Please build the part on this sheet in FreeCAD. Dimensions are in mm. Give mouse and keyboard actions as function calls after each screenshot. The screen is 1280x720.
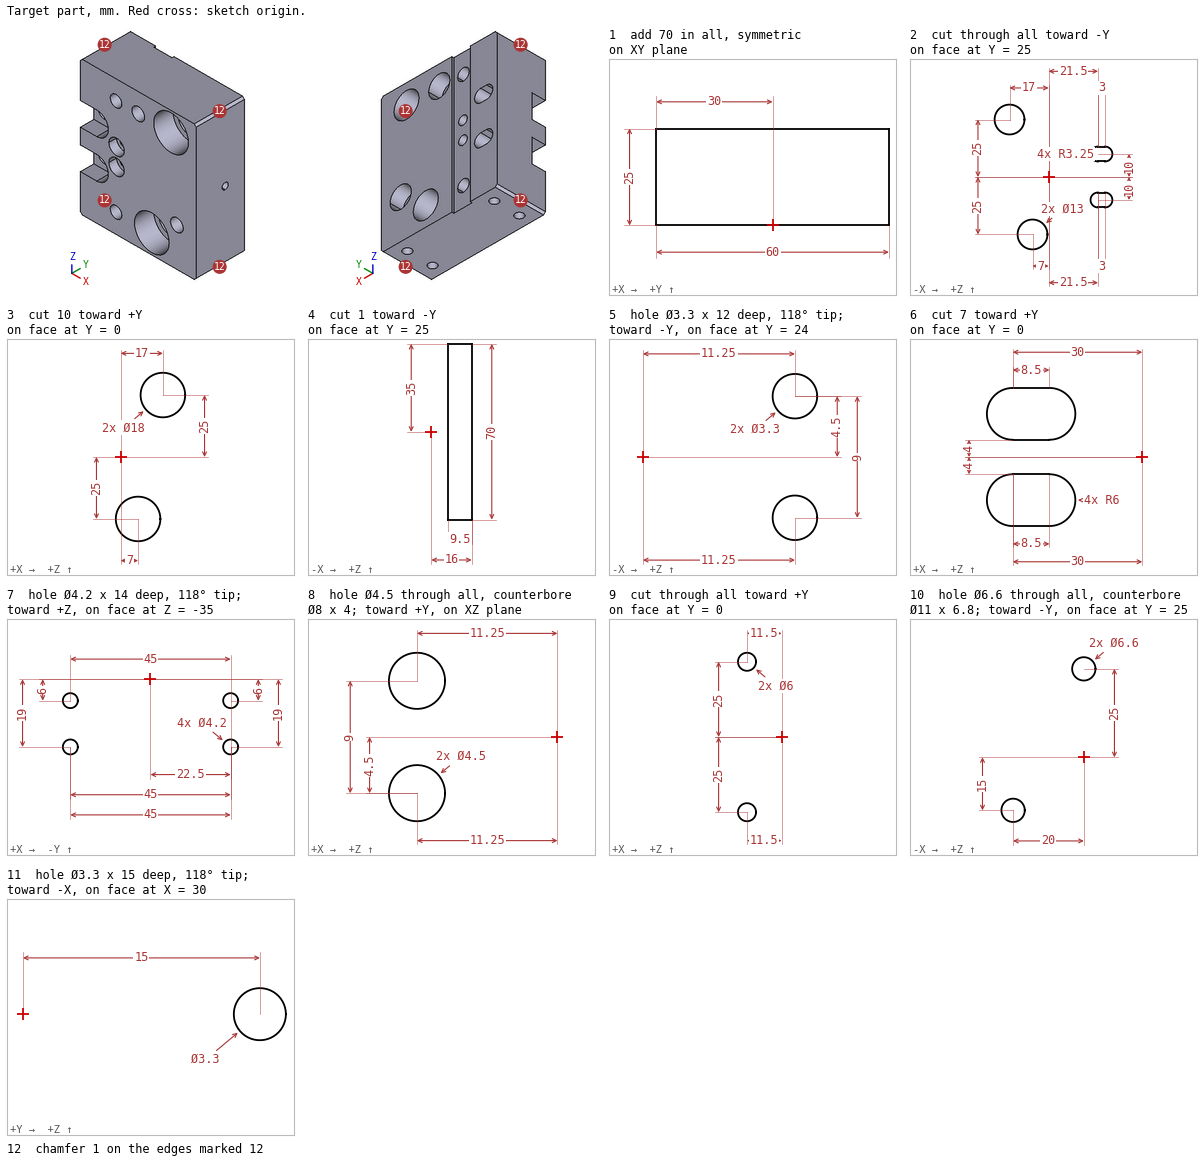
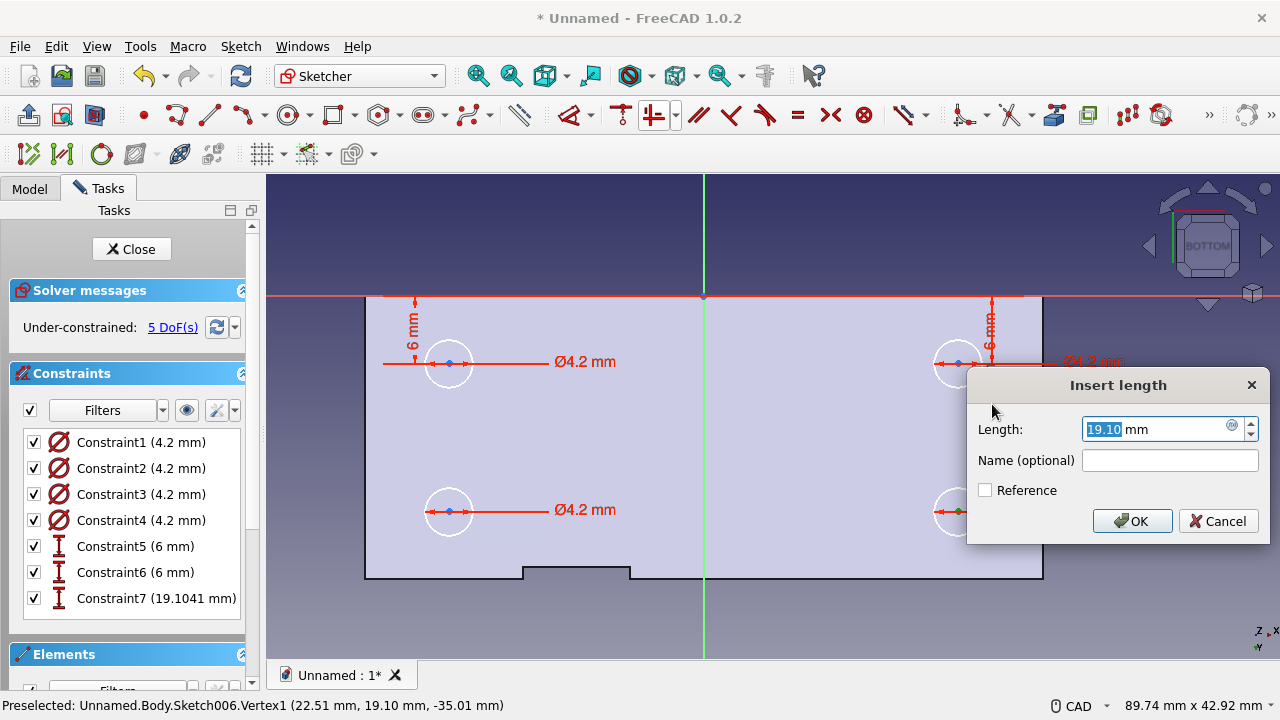
text(19)
key(Return)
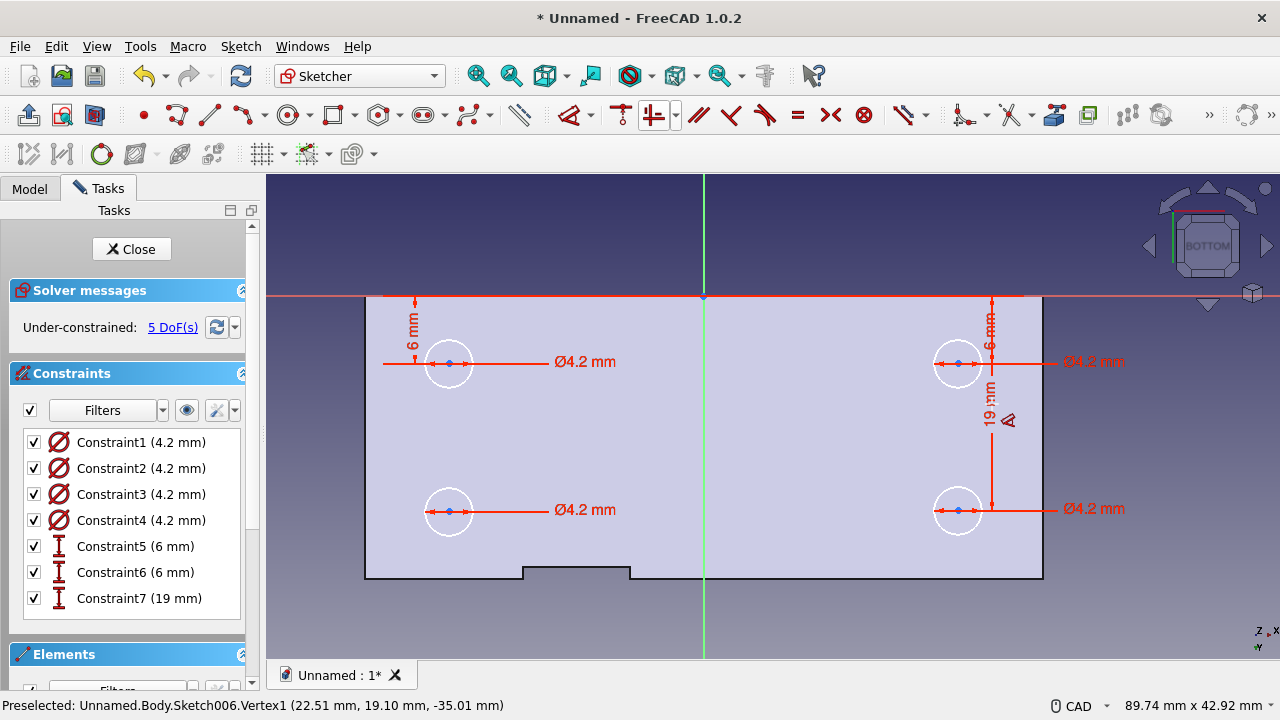
click(449, 512)
click(415, 404)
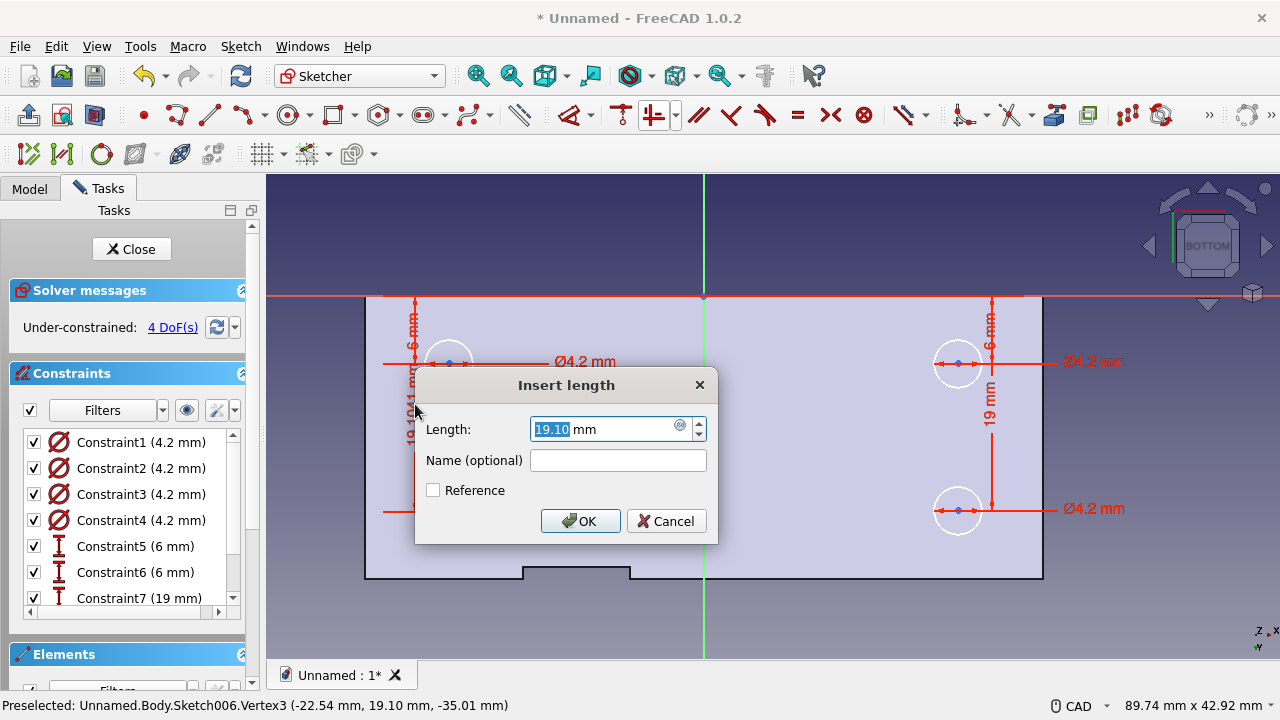
text(19)
key(Return)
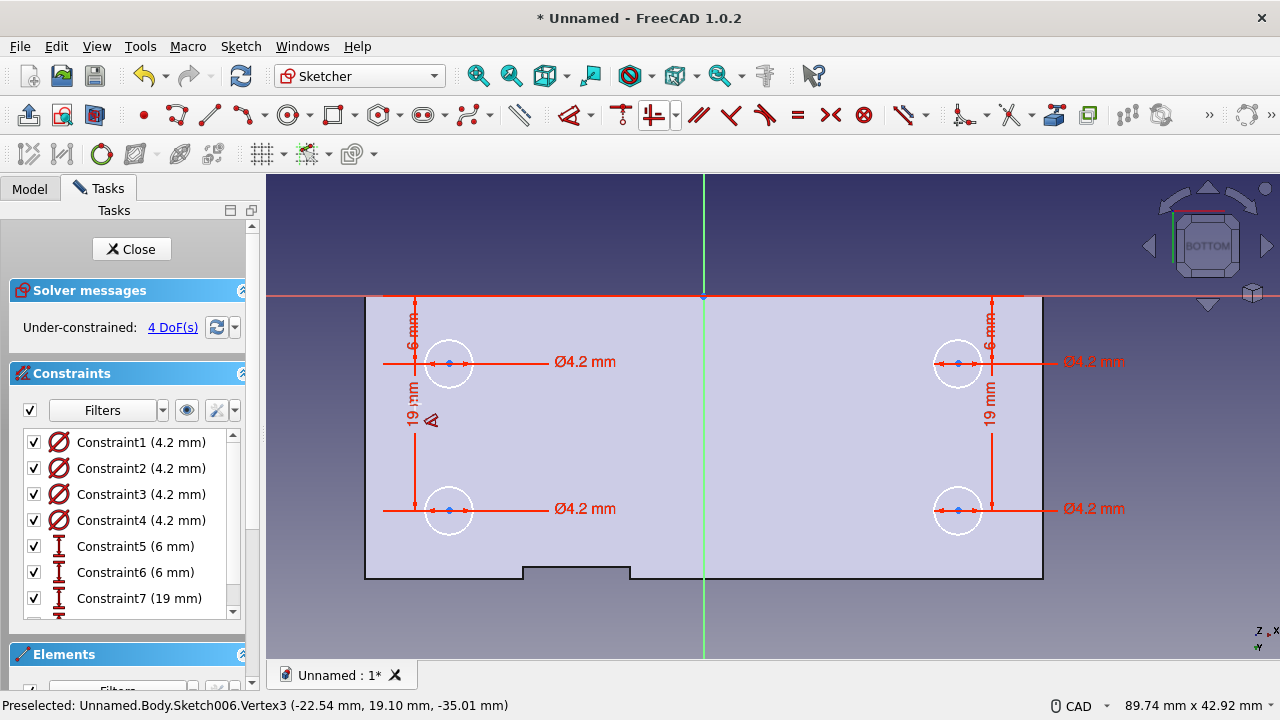
click(958, 511)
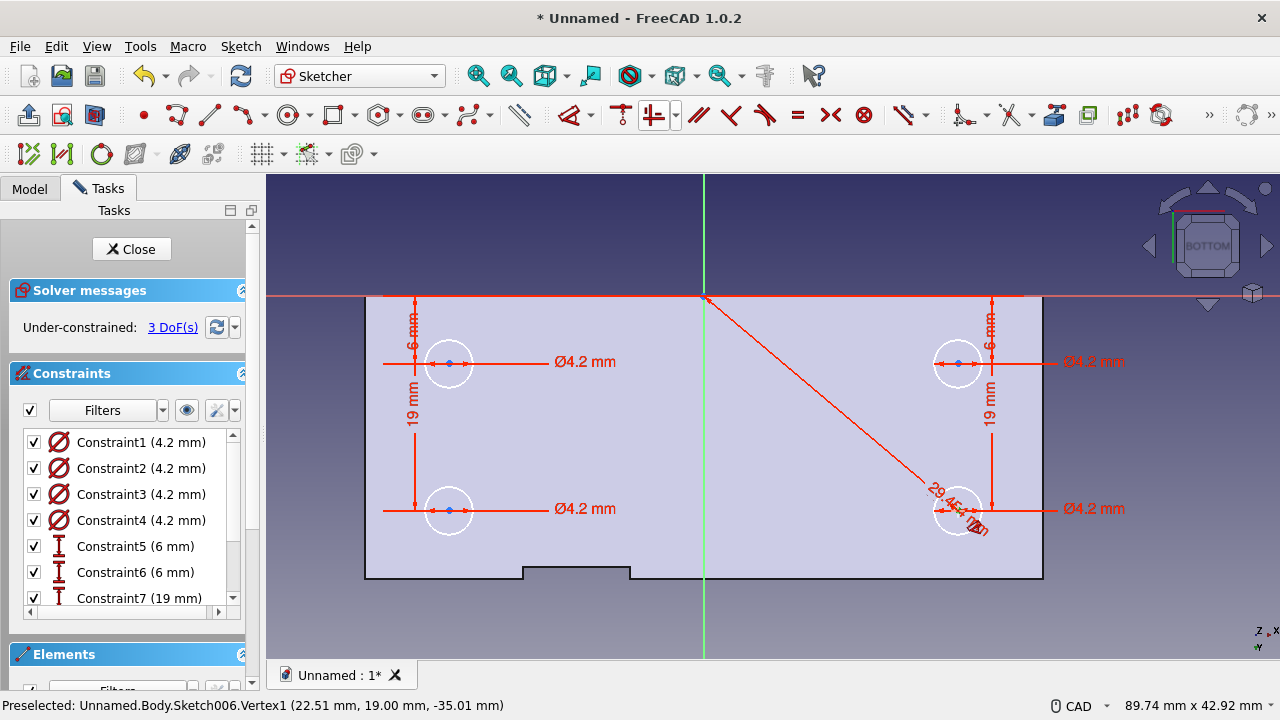
click(449, 511)
click(586, 545)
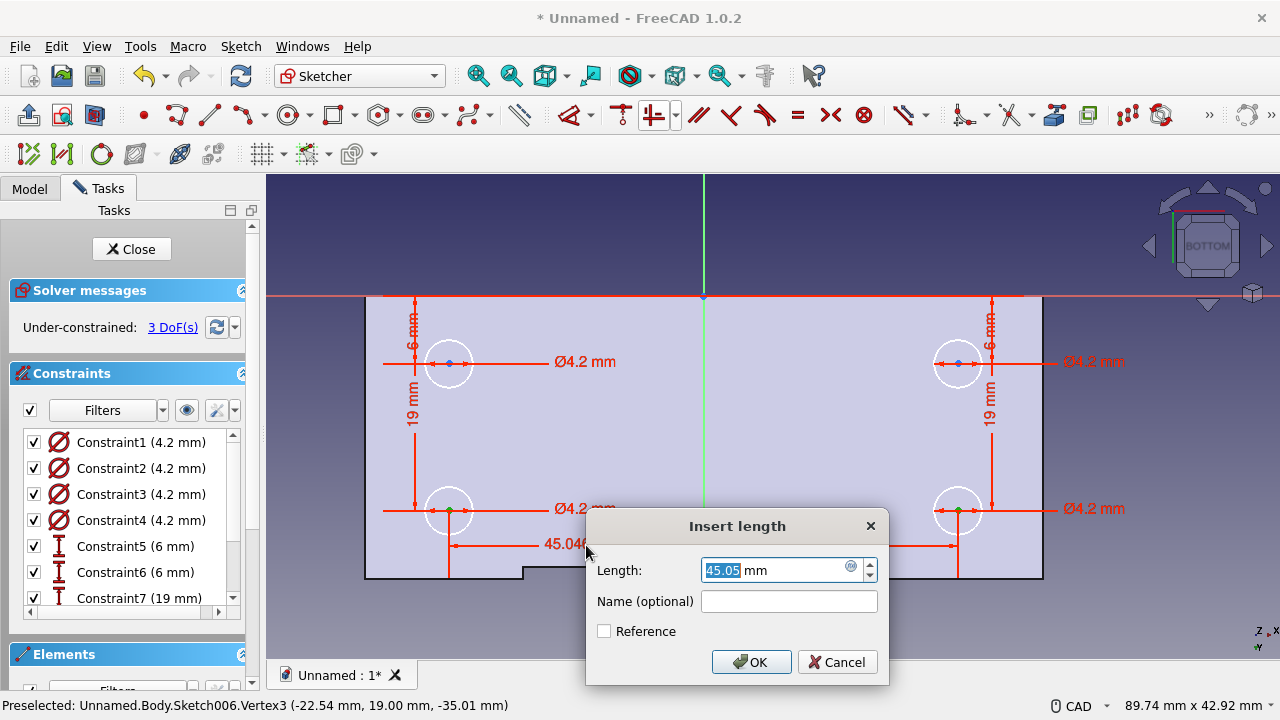
text(45)
key(Return)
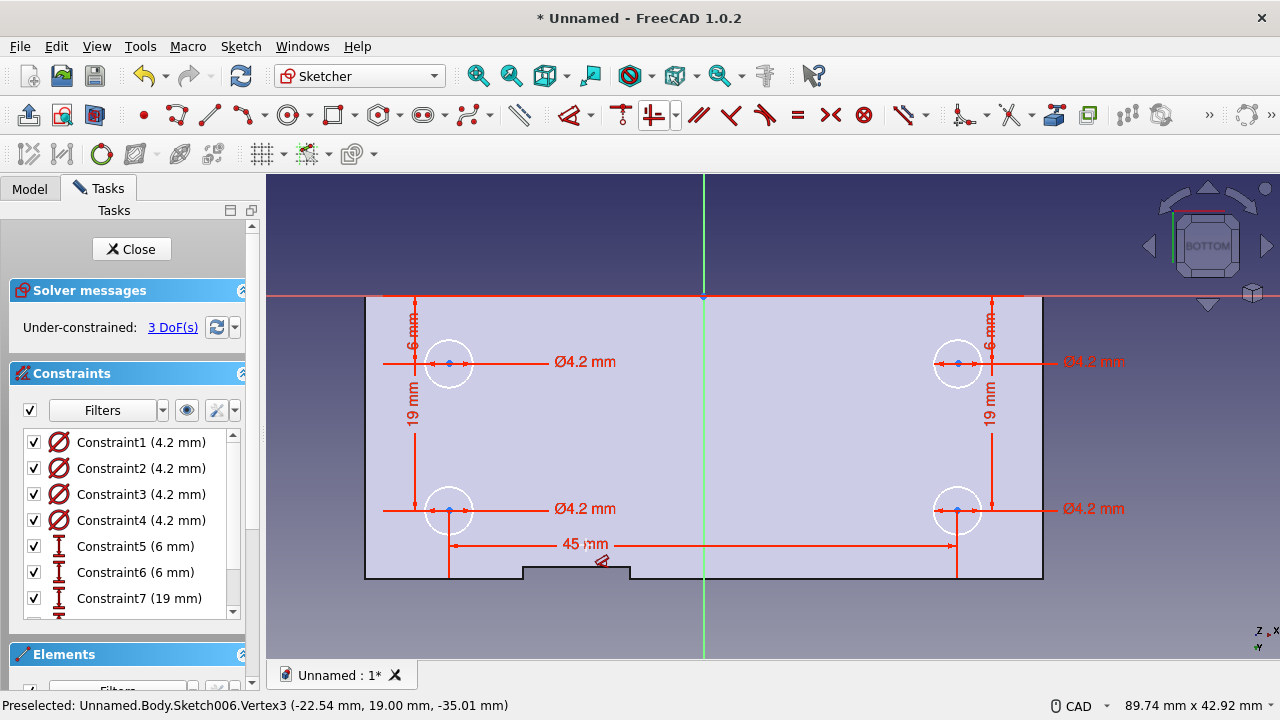
click(958, 364)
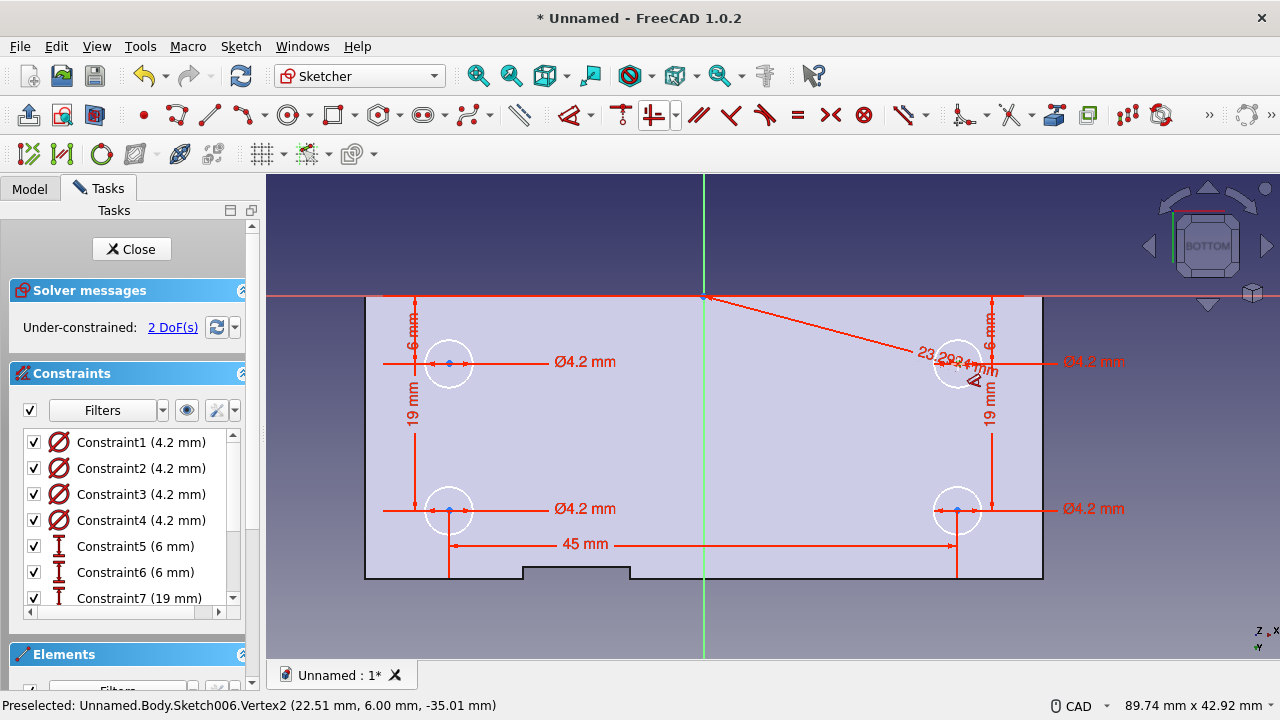
click(449, 511)
click(821, 545)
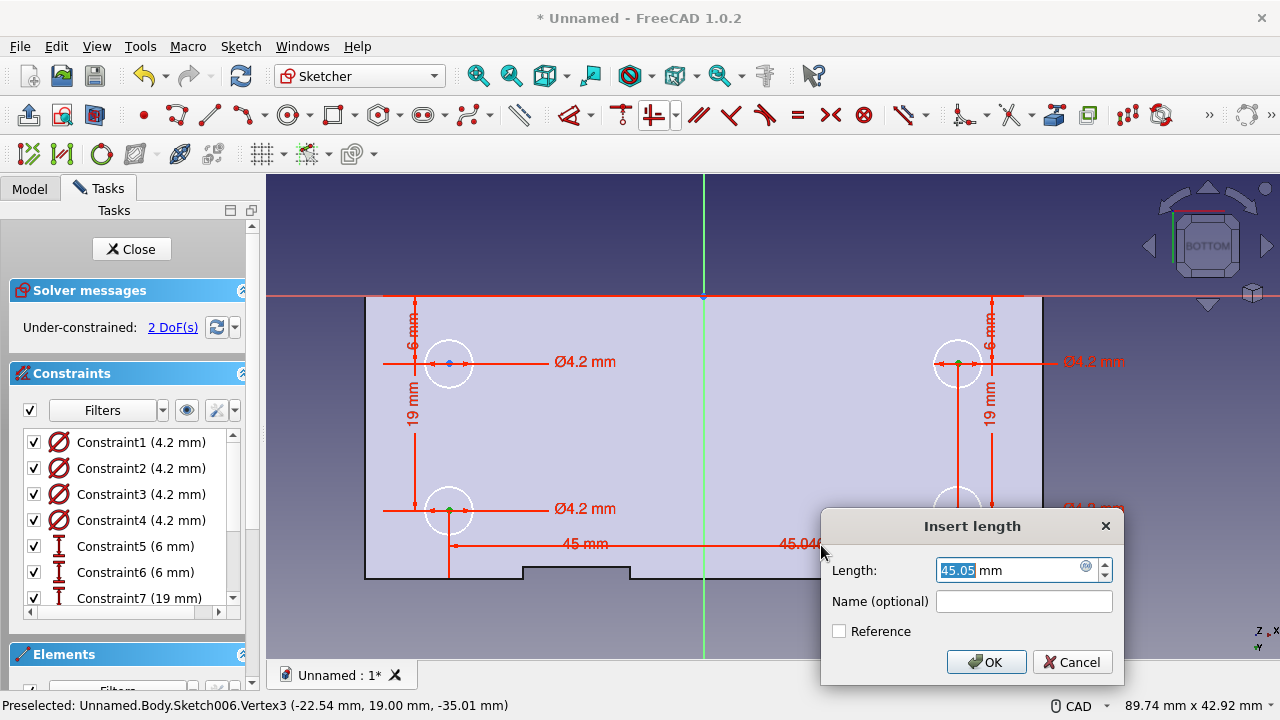
text(45)
key(Return)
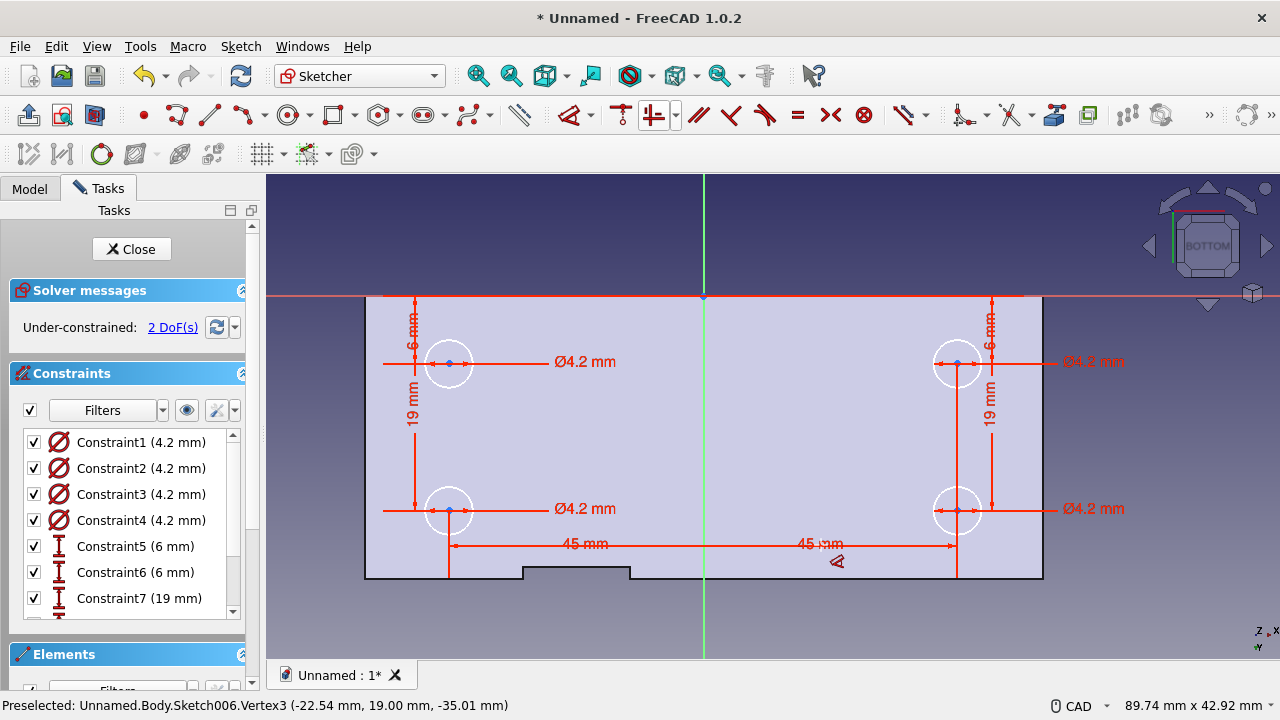
click(957, 364)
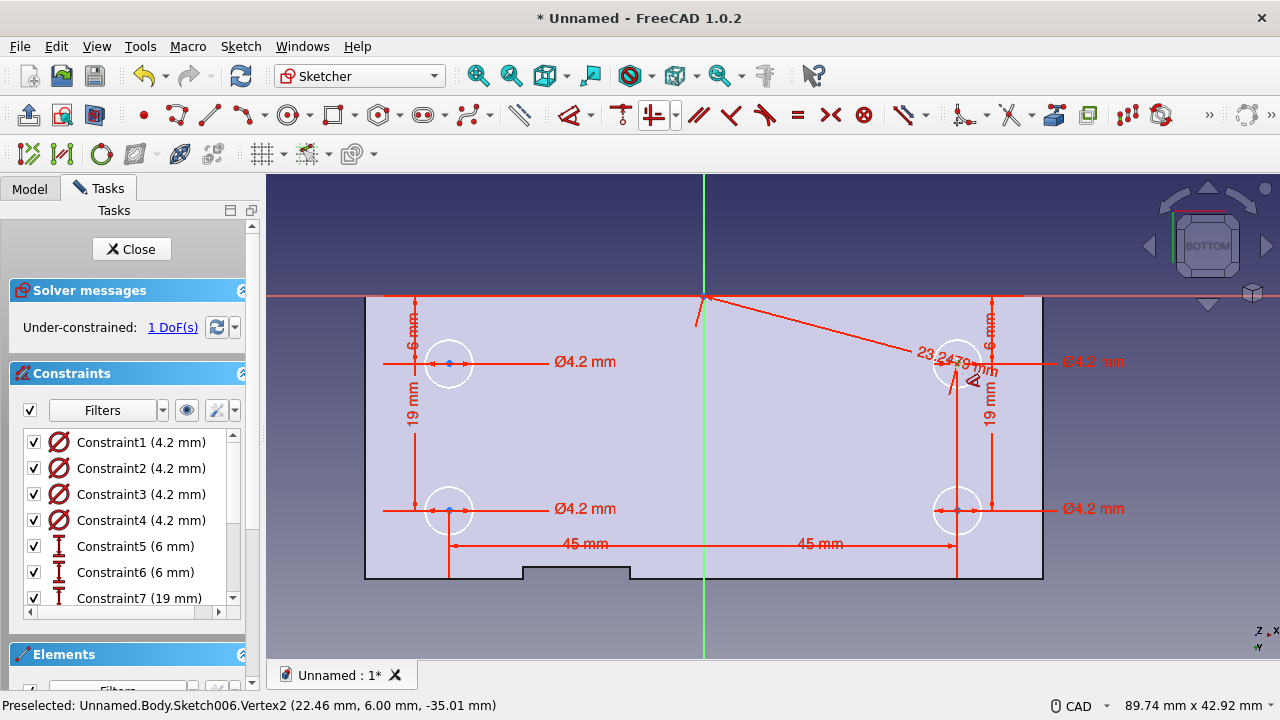
click(449, 364)
click(586, 330)